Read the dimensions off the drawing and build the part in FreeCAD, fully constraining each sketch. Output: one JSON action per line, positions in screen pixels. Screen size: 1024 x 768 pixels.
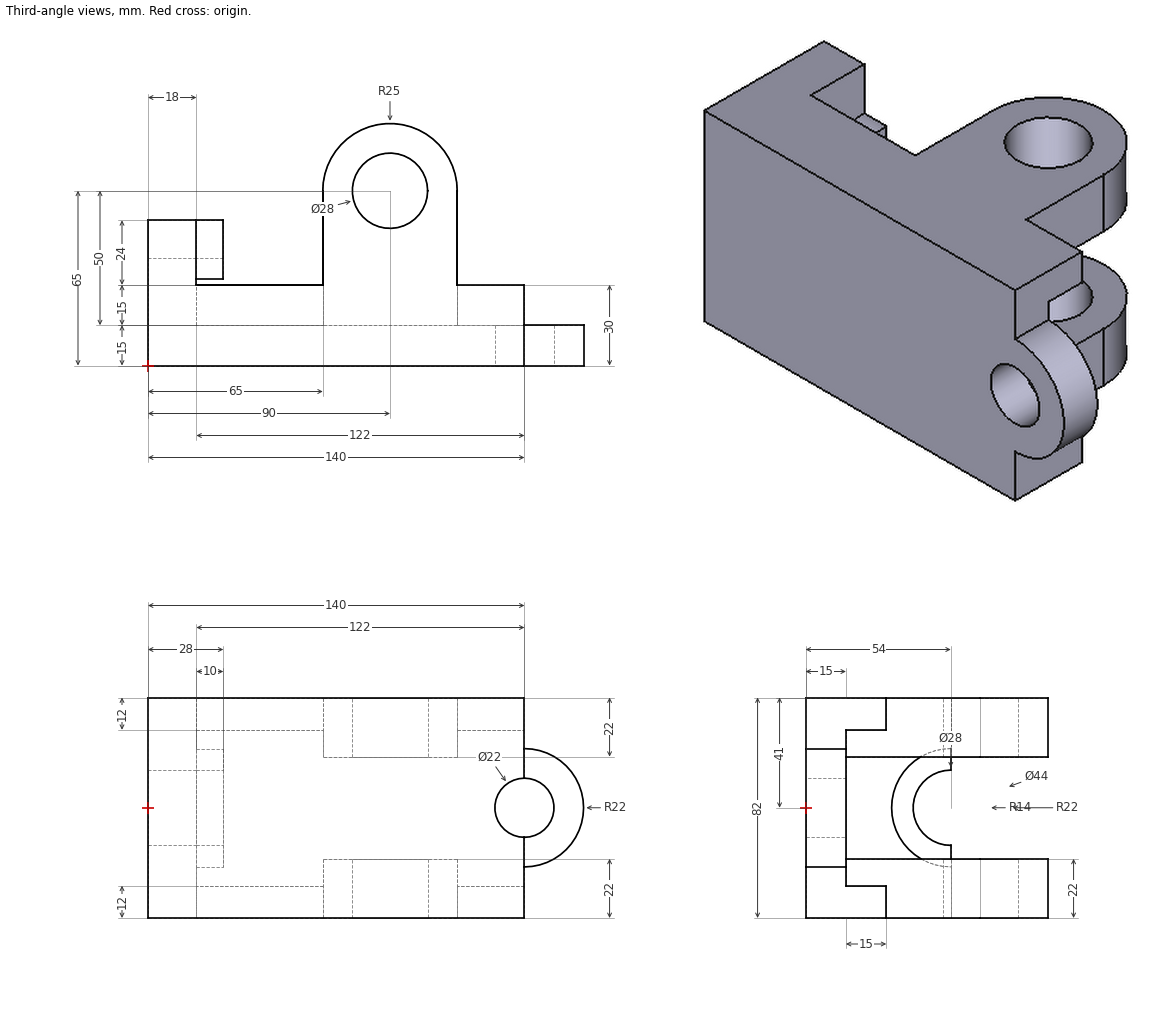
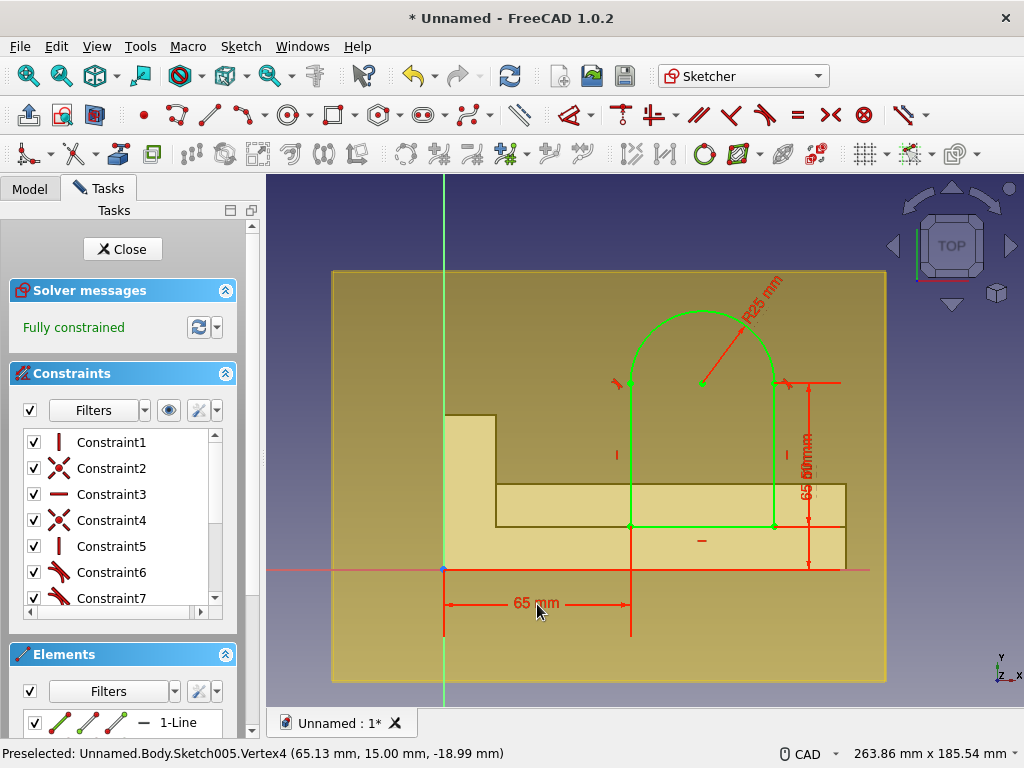
{"action": "left_click", "coordinate": [123, 249]}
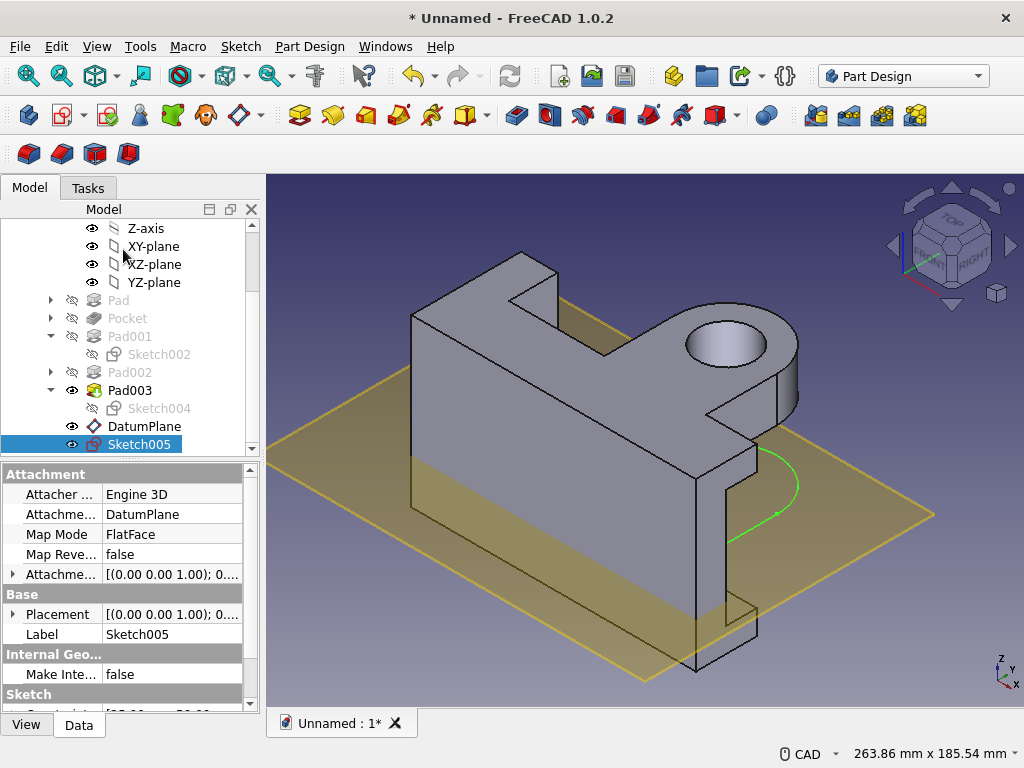
{"action": "left_click", "coordinate": [300, 116]}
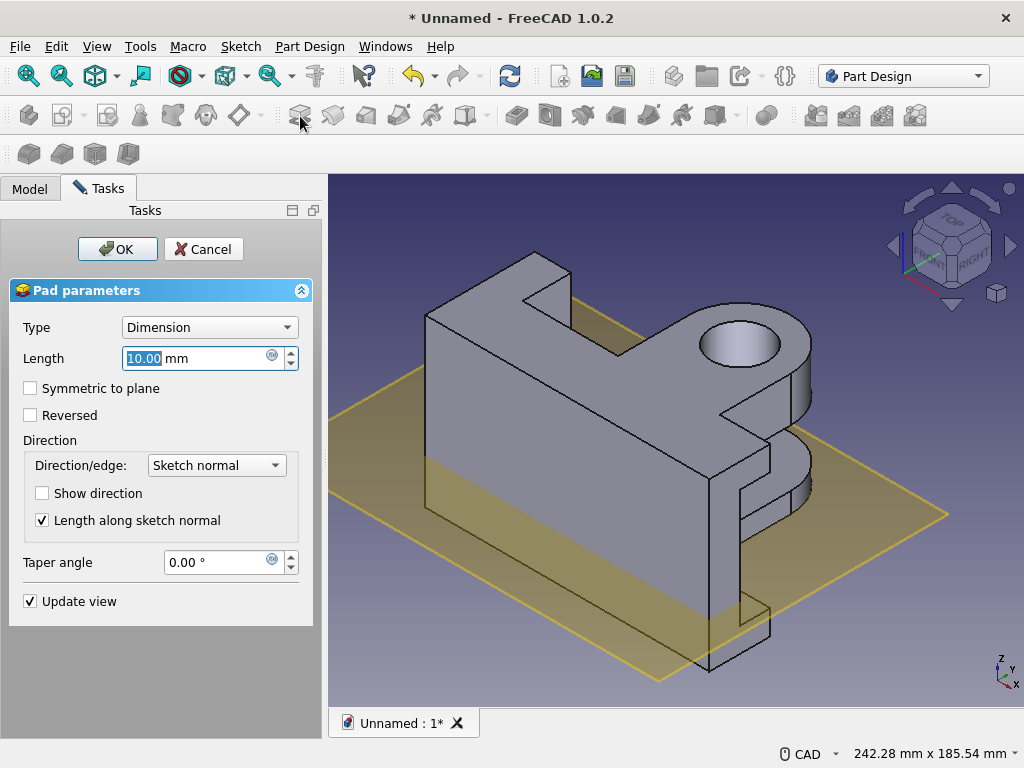
{"action": "type", "text": "22"}
{"action": "key", "text": "Tab"}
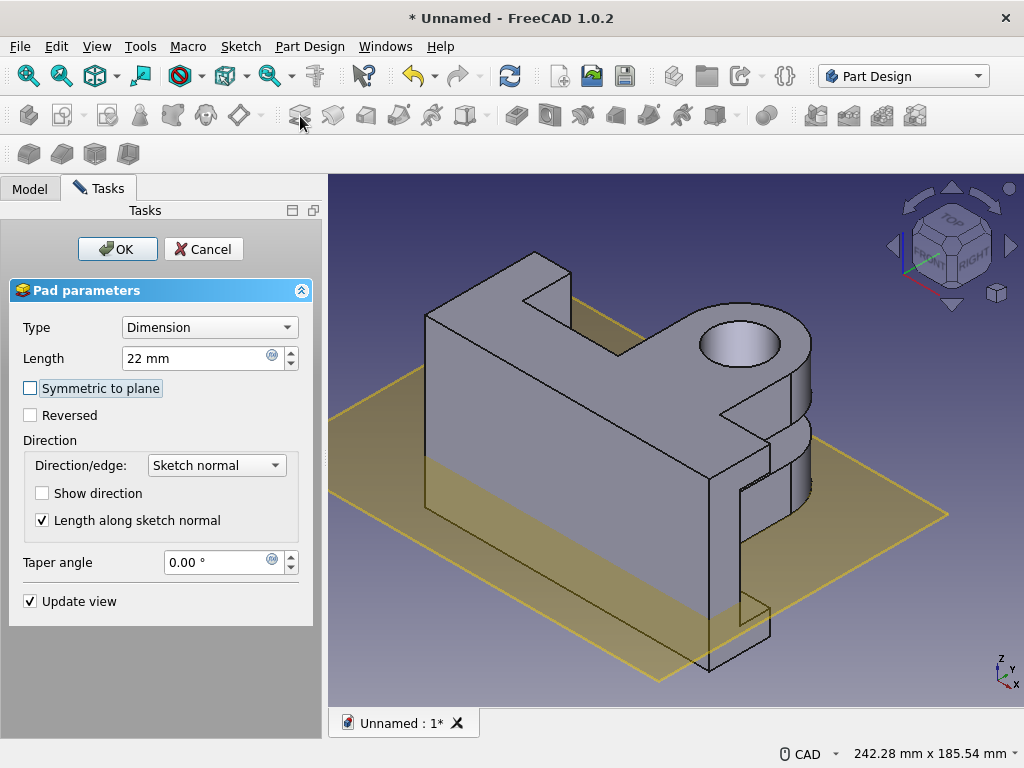
{"action": "left_click", "coordinate": [31, 415]}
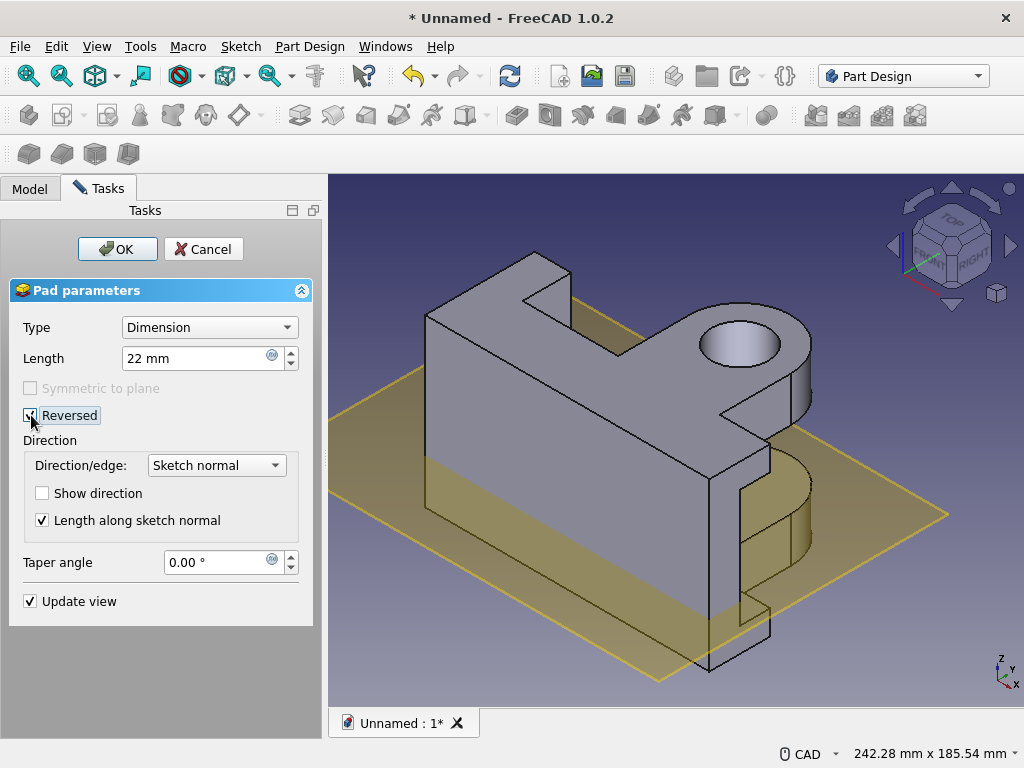
{"action": "left_click", "coordinate": [118, 249]}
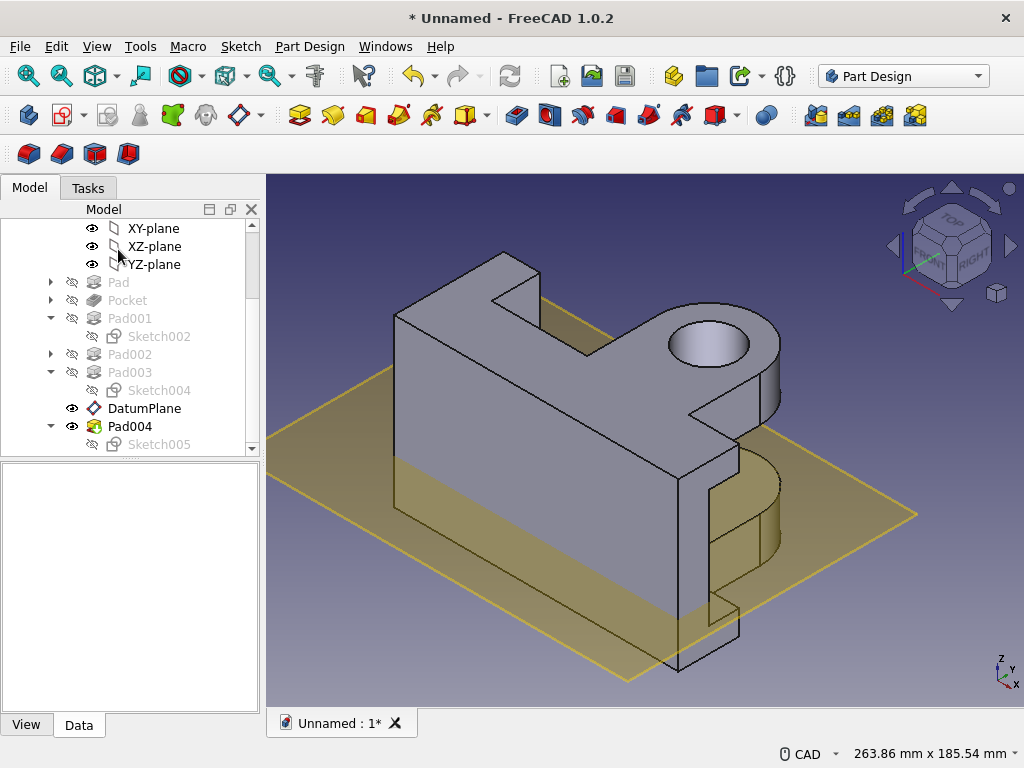
{"action": "left_click", "coordinate": [117, 408]}
{"action": "key", "text": "space"}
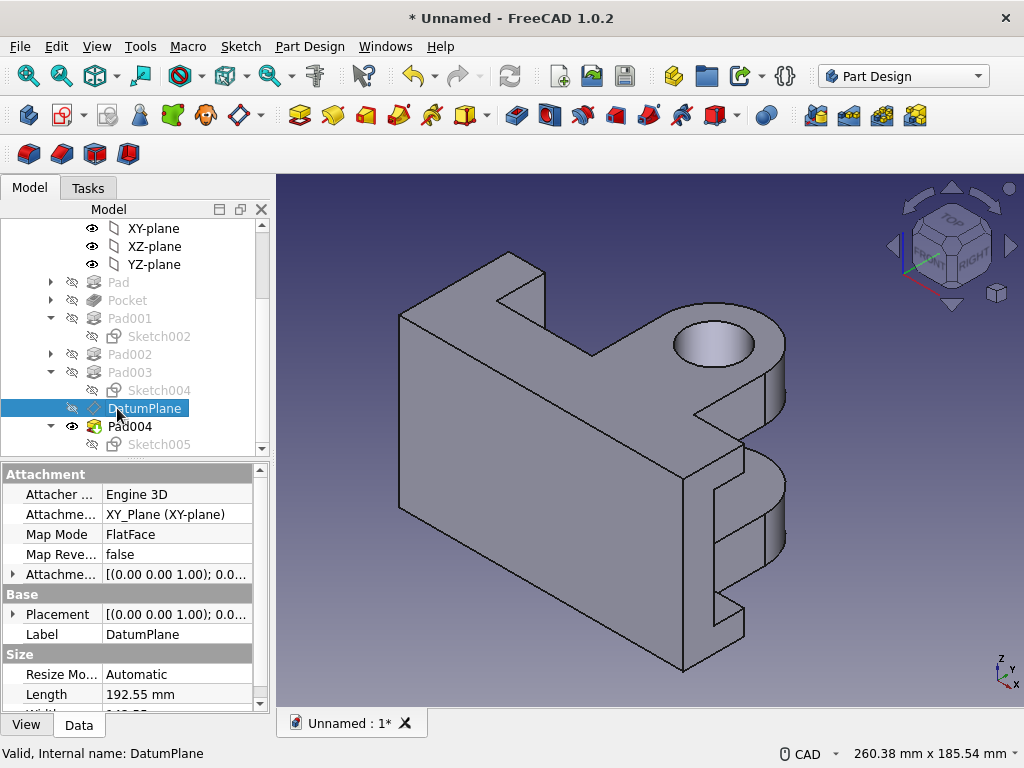
{"action": "left_click", "coordinate": [725, 495]}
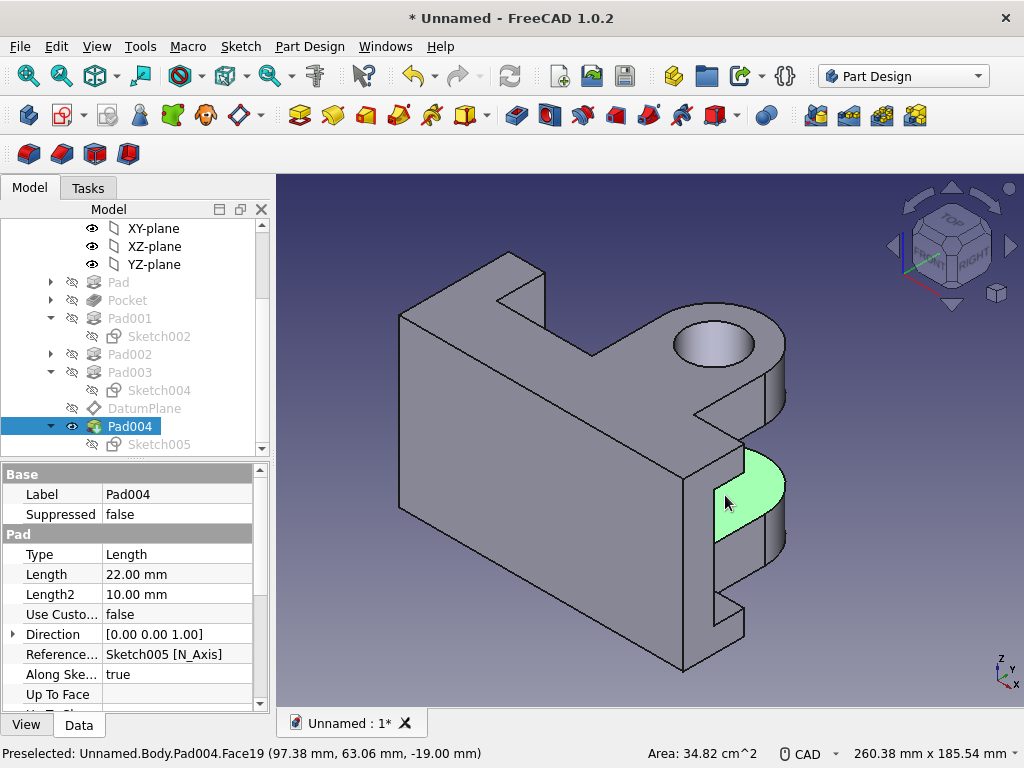
{"action": "left_click", "coordinate": [62, 116]}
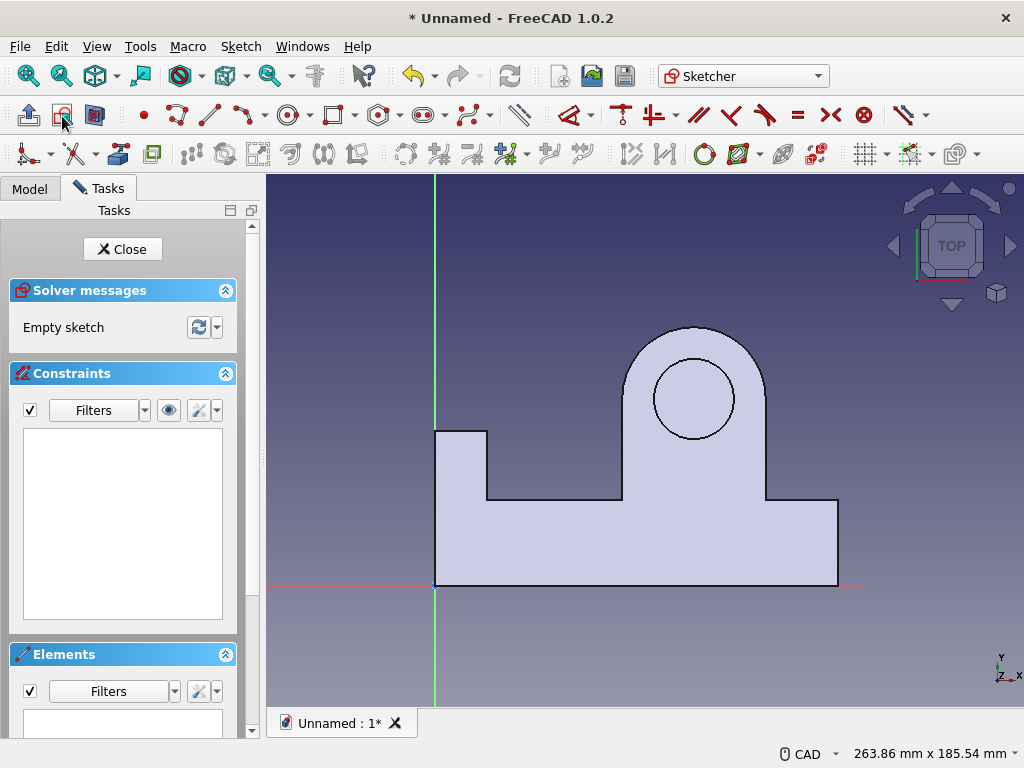
{"action": "scroll", "coordinate": [732, 385], "scroll_direction": "up", "scroll_amount": 7}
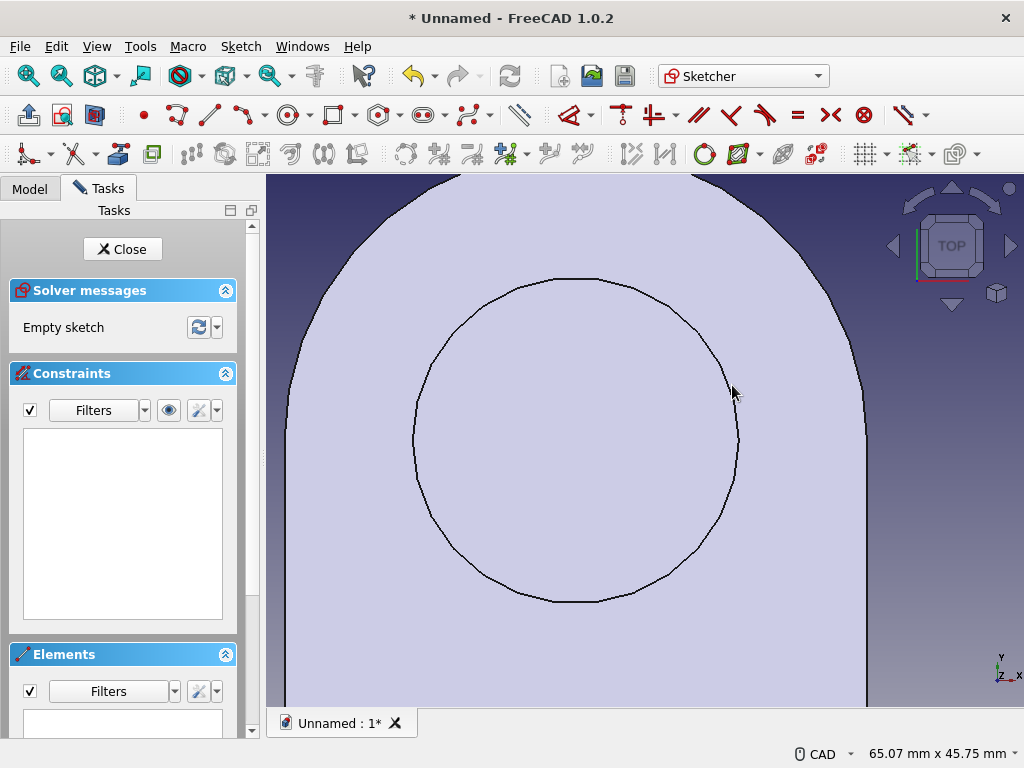
{"action": "key", "text": "g c"}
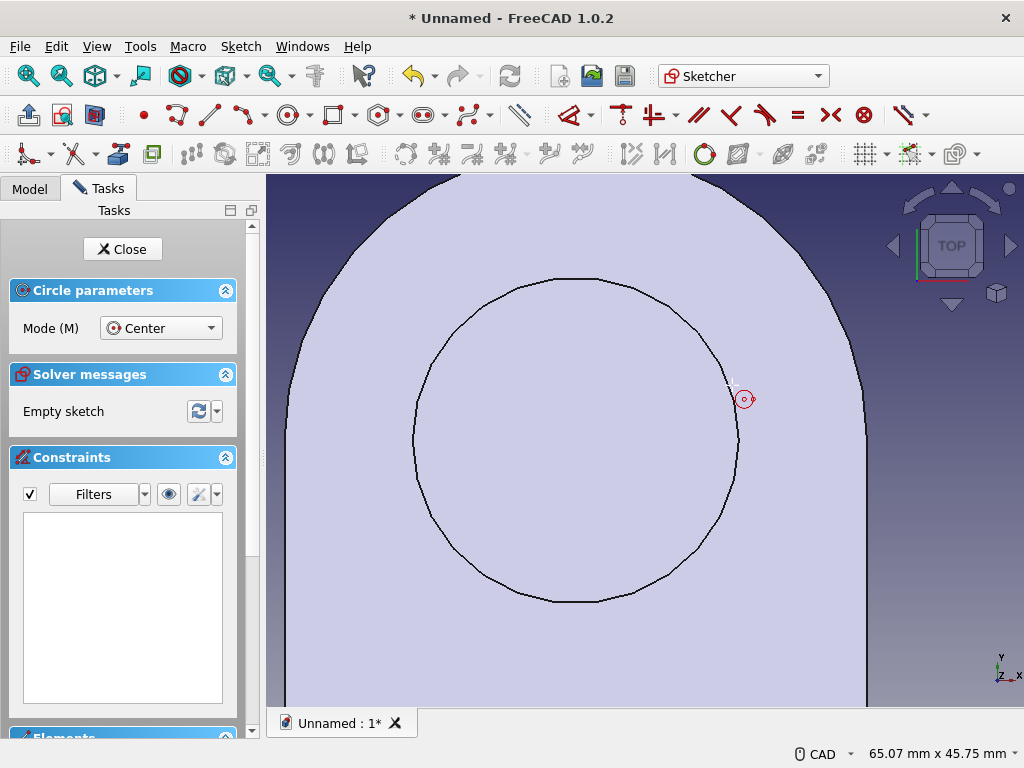
{"action": "left_click", "coordinate": [576, 441]}
{"action": "left_click", "coordinate": [691, 325]}
{"action": "key", "text": "Escape"}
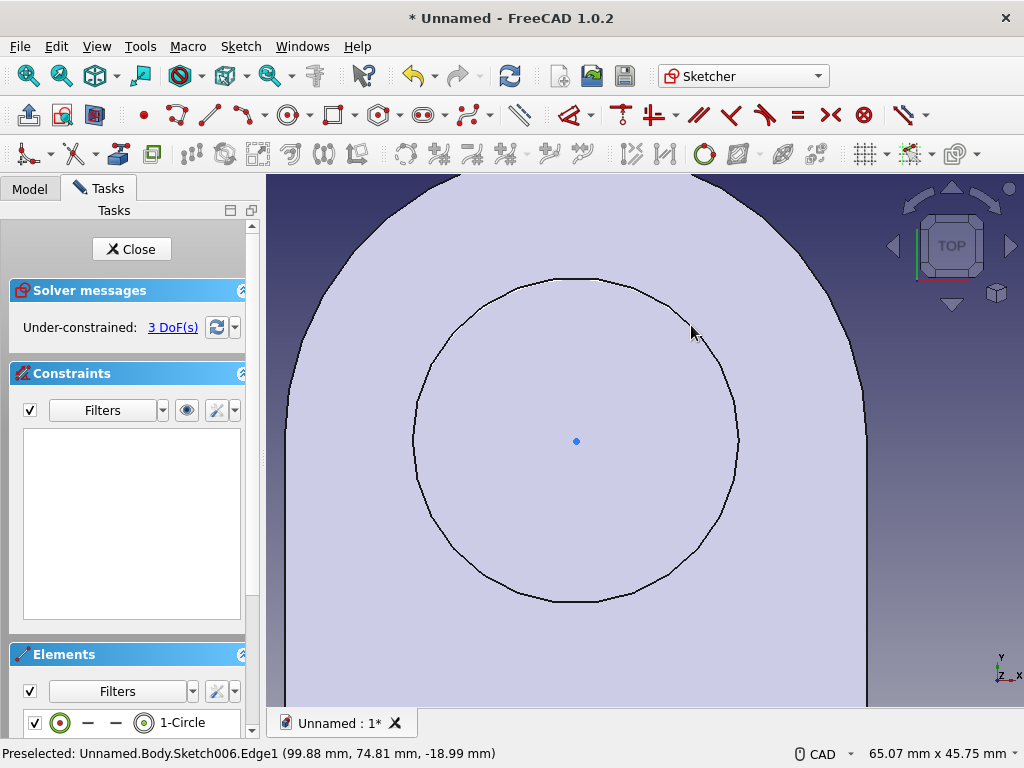
{"action": "key", "text": "d"}